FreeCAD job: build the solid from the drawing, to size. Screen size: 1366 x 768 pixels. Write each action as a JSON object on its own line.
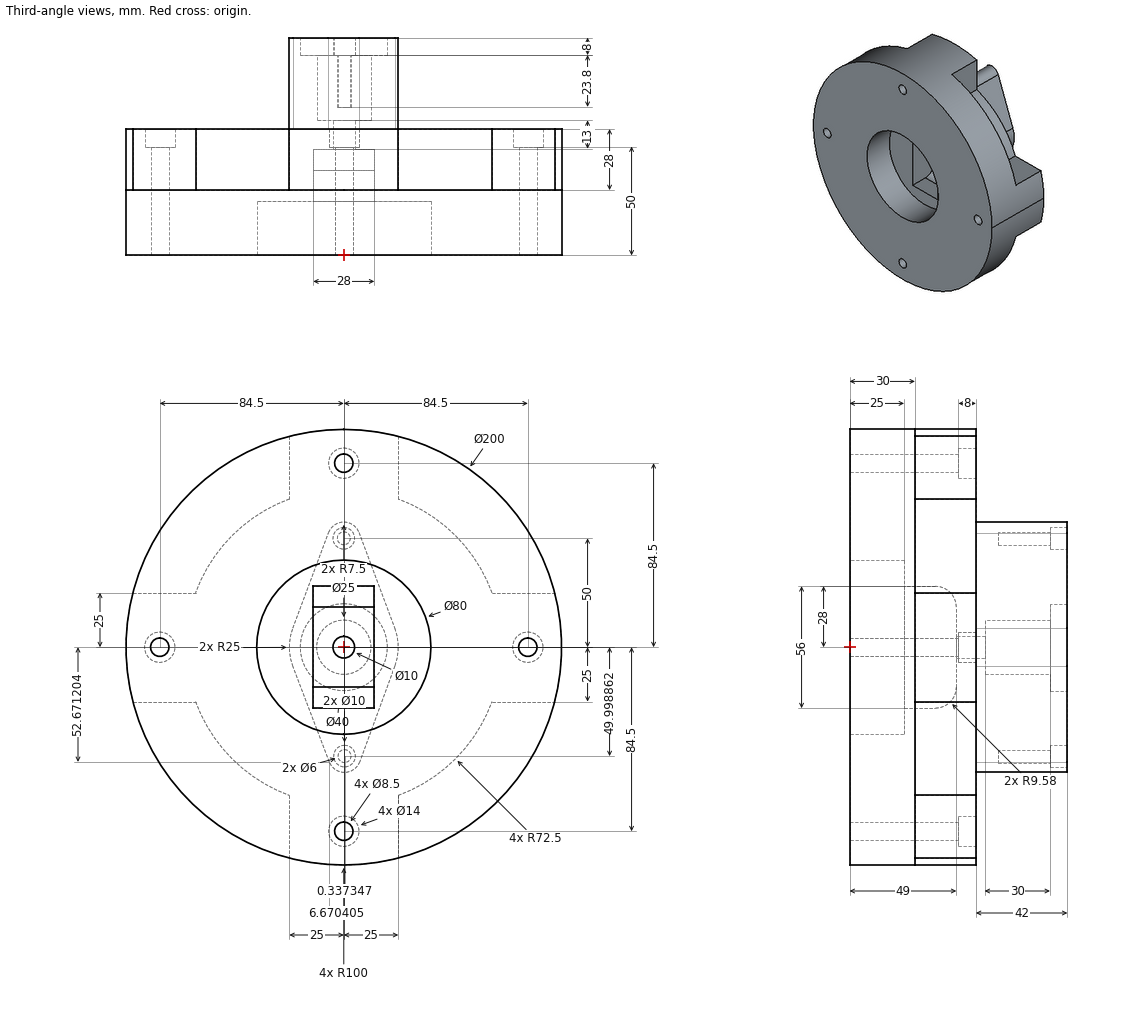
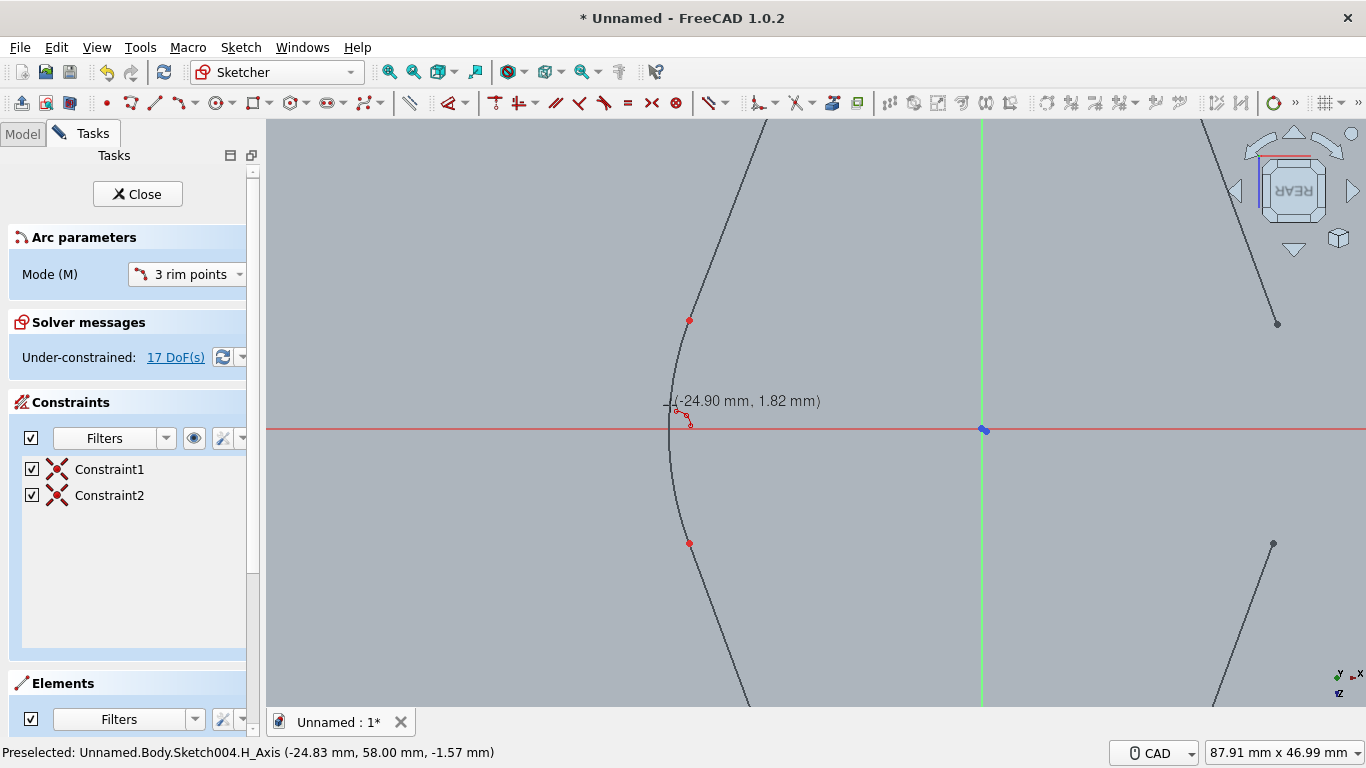
{"action": "scroll", "coordinate": [671, 408], "scroll_direction": "down", "scroll_amount": 7}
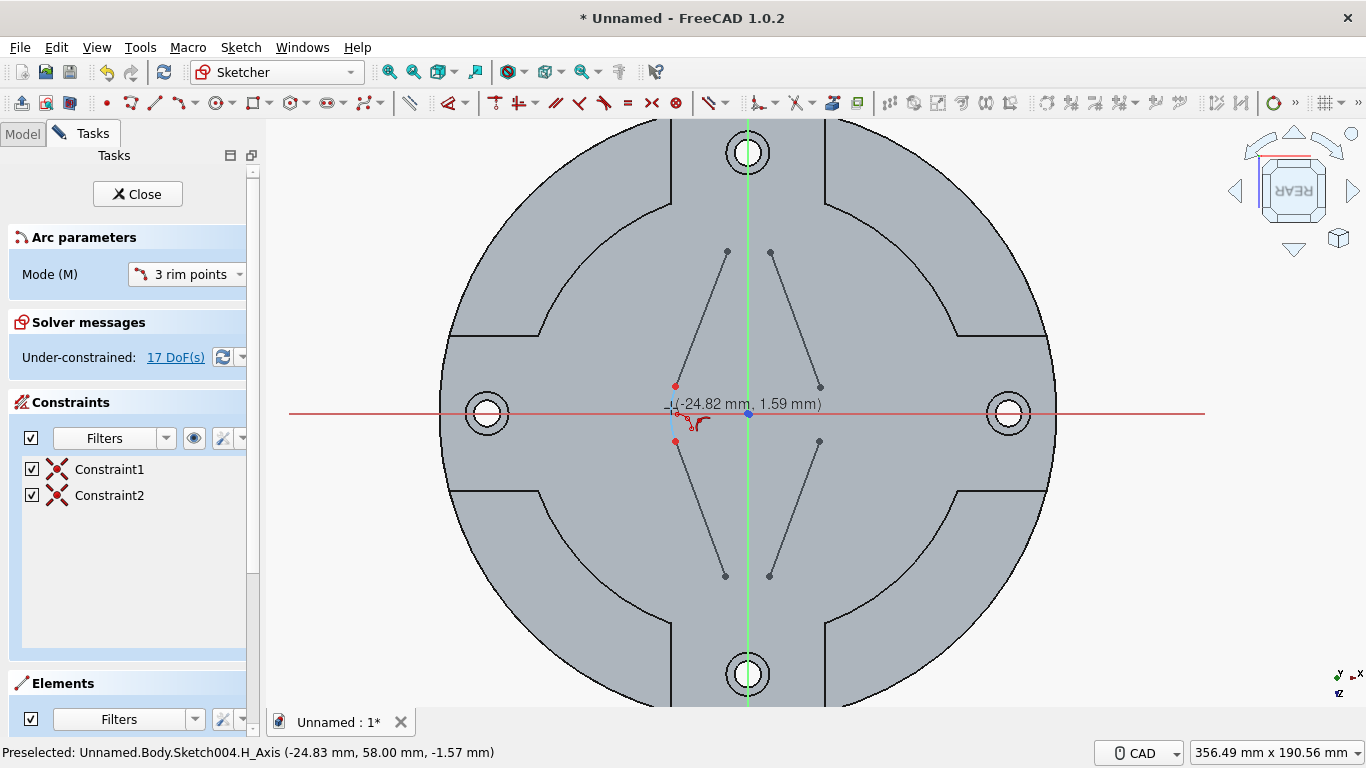
{"action": "left_click", "coordinate": [726, 577]}
{"action": "left_click", "coordinate": [770, 577]}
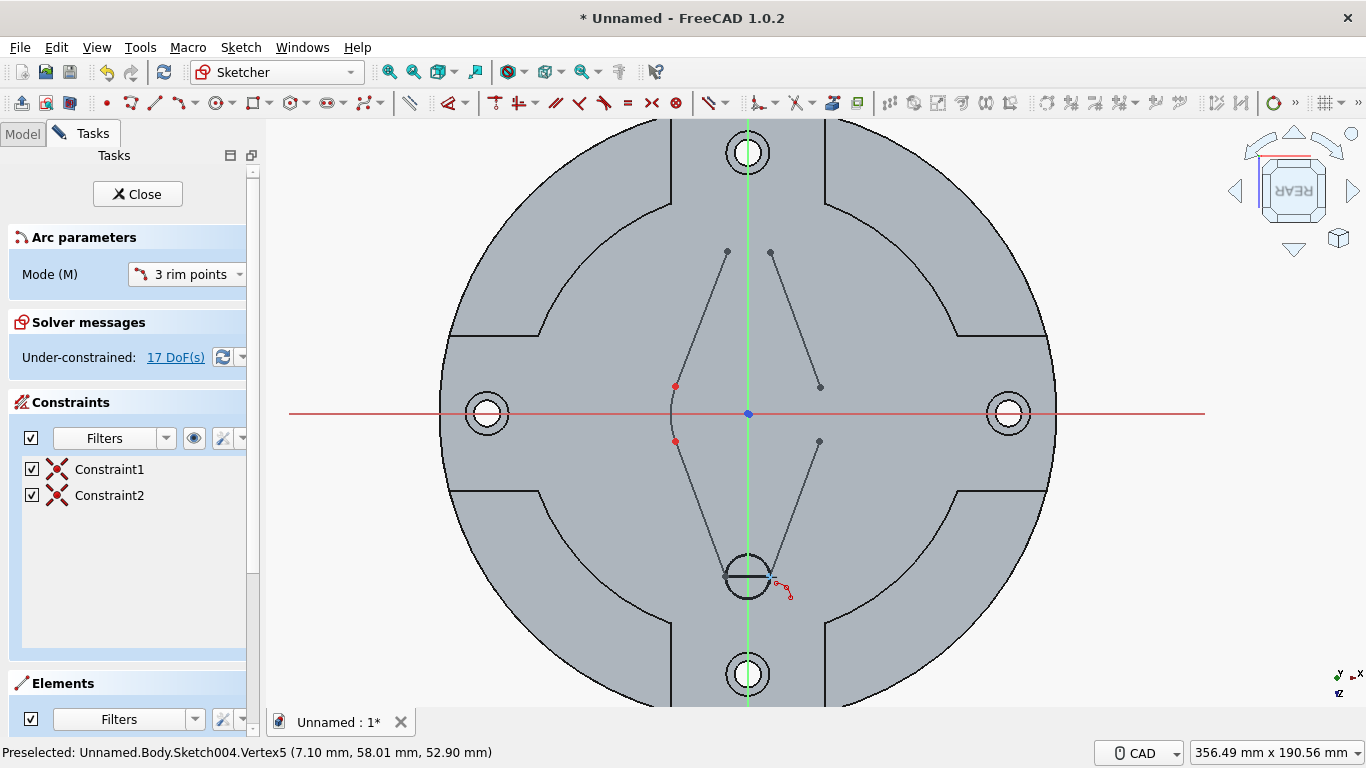
{"action": "scroll", "coordinate": [737, 588], "scroll_direction": "up", "scroll_amount": 2}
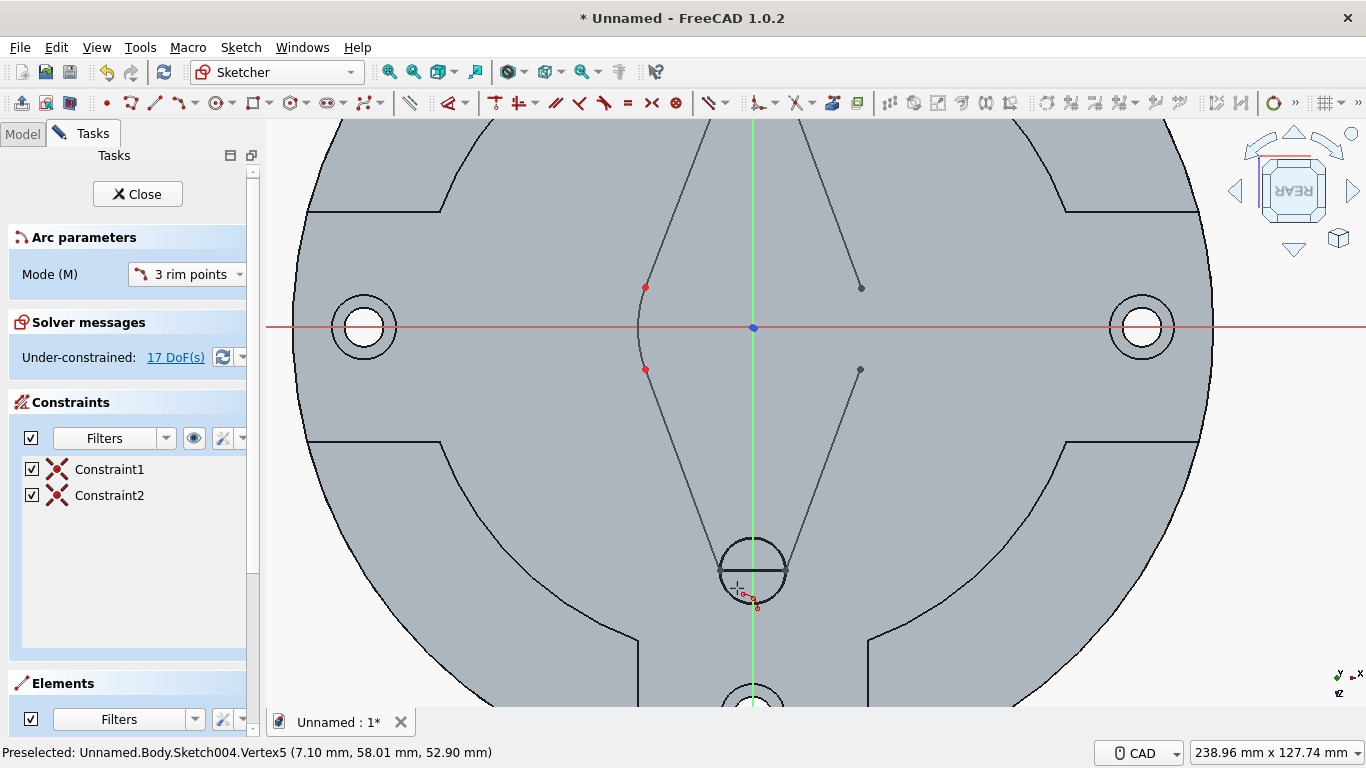
{"action": "left_click", "coordinate": [737, 588]}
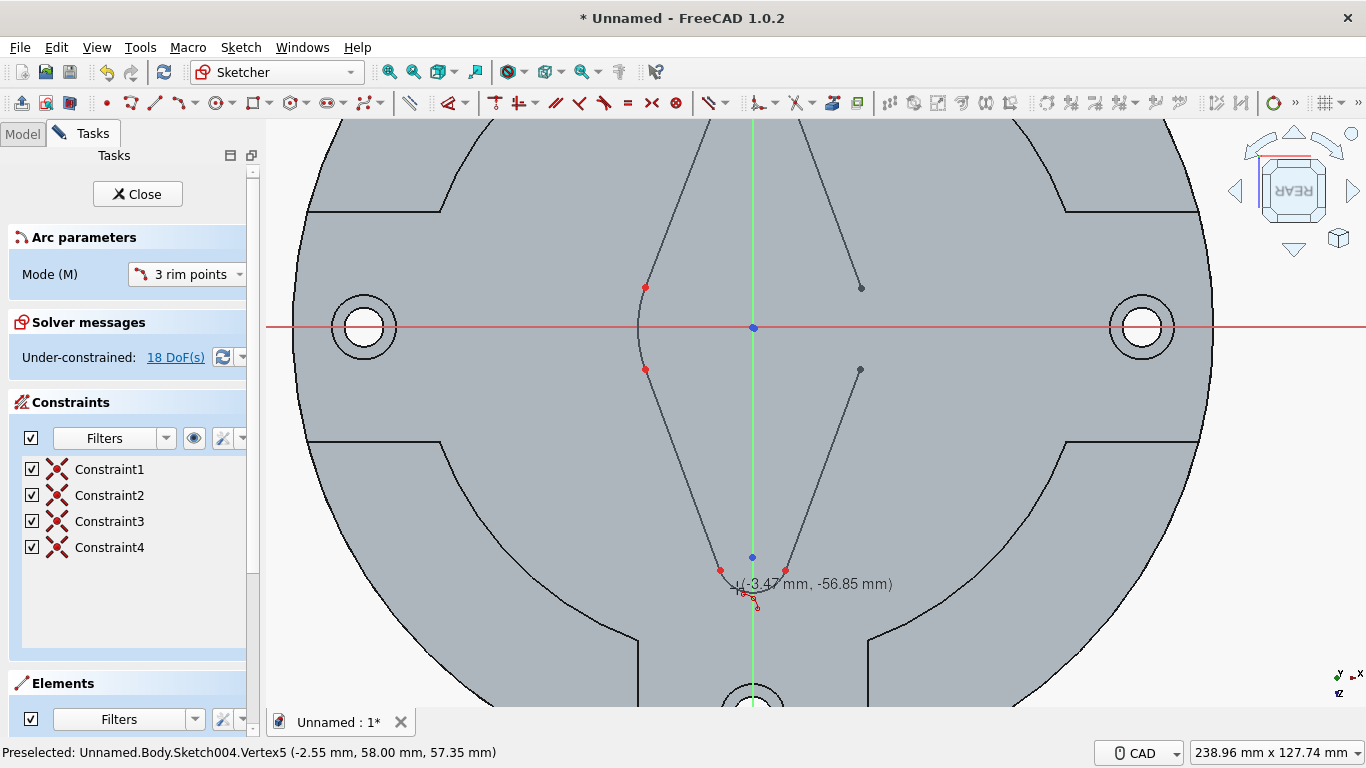
{"action": "left_click", "coordinate": [860, 369]}
{"action": "left_click", "coordinate": [862, 289]}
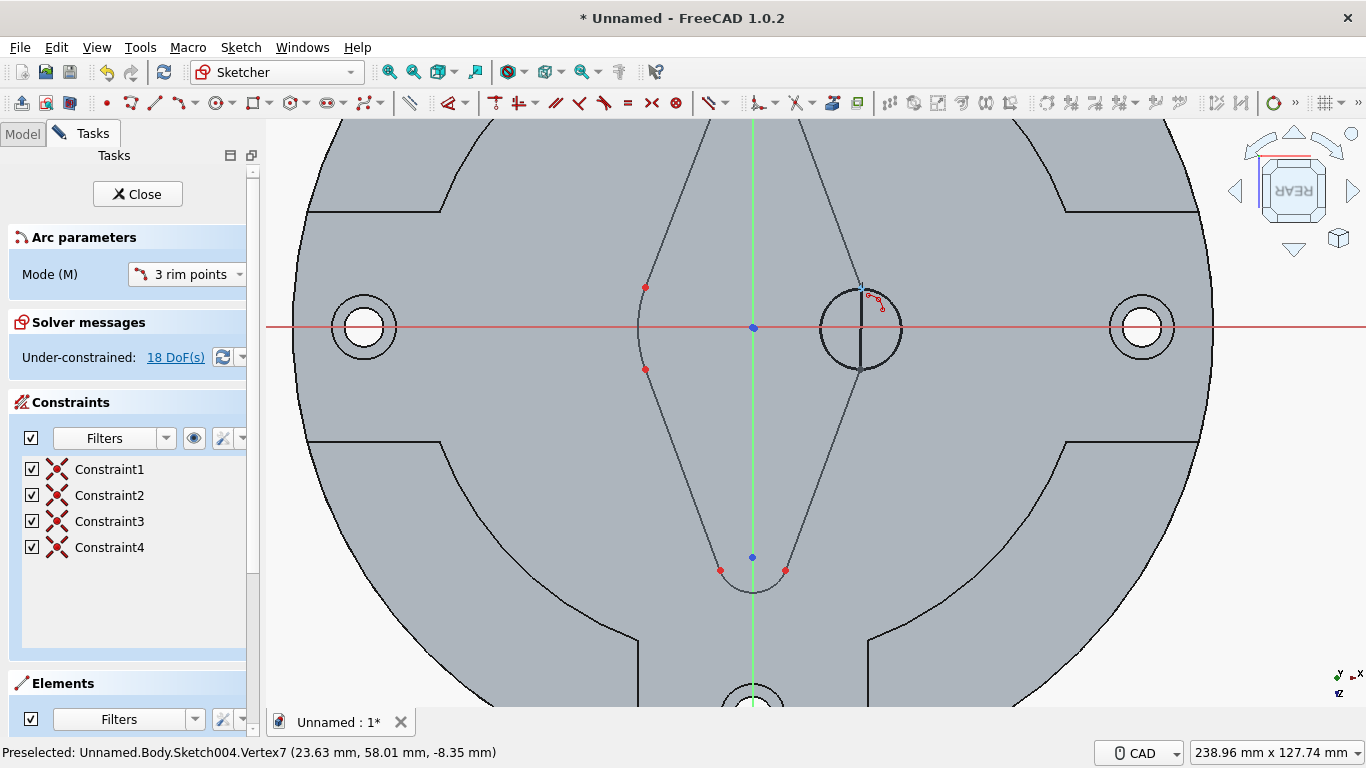
{"action": "scroll", "coordinate": [868, 336], "scroll_direction": "up", "scroll_amount": 5}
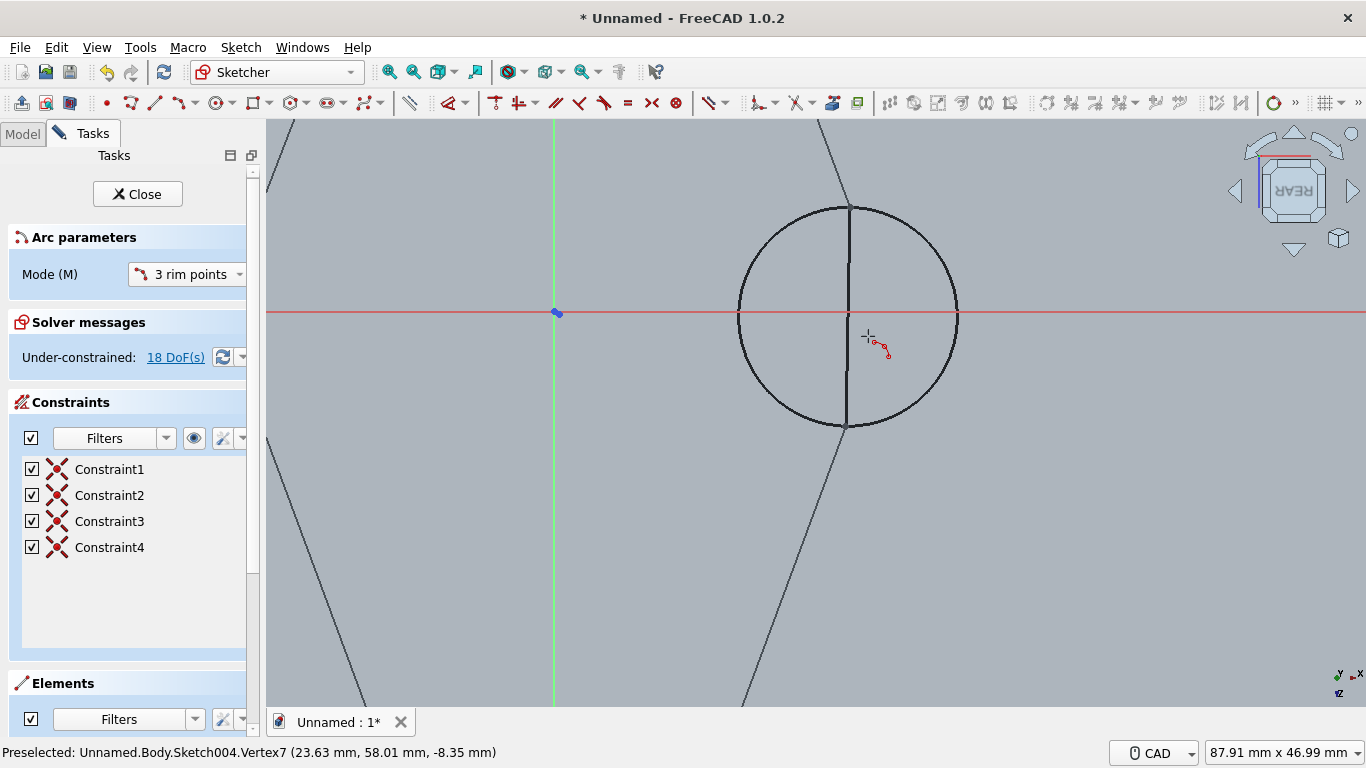
{"action": "left_click", "coordinate": [866, 335]}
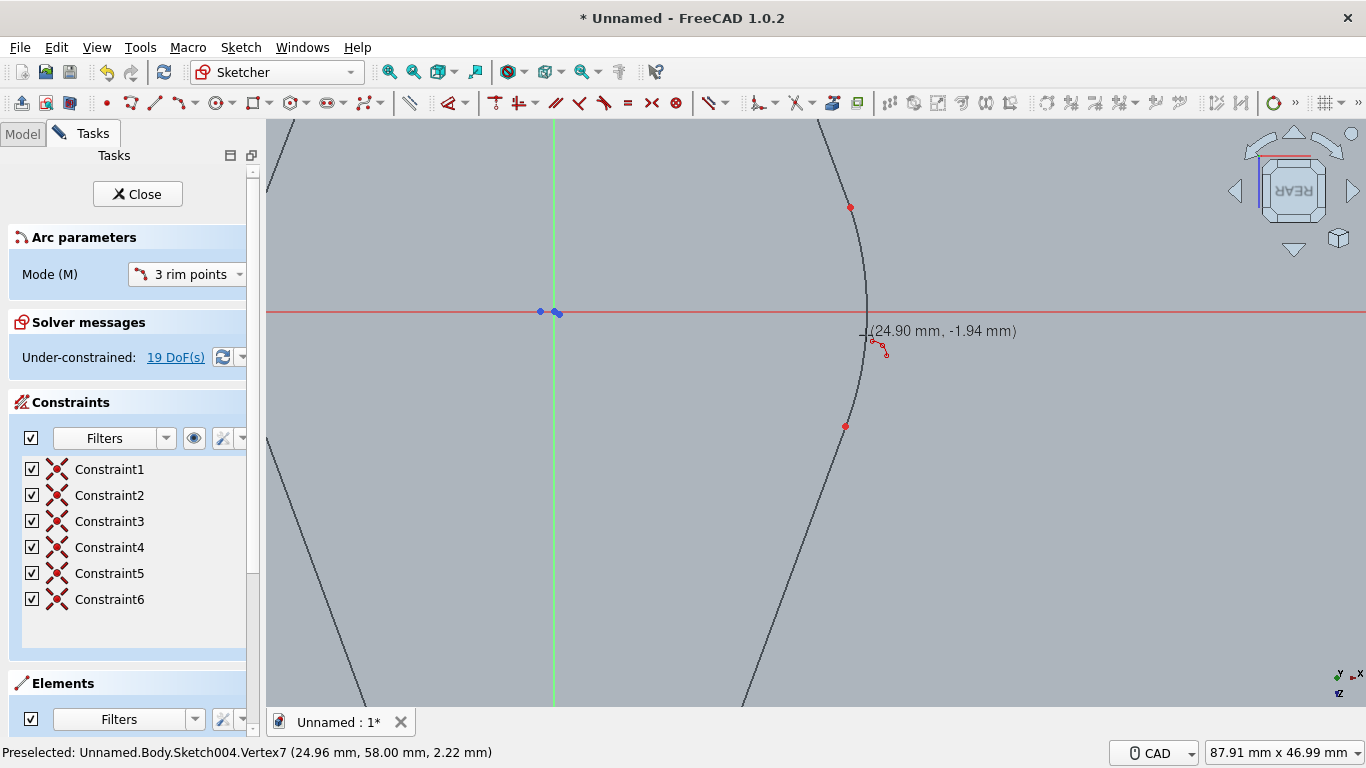
{"action": "scroll", "coordinate": [811, 446], "scroll_direction": "down", "scroll_amount": 7}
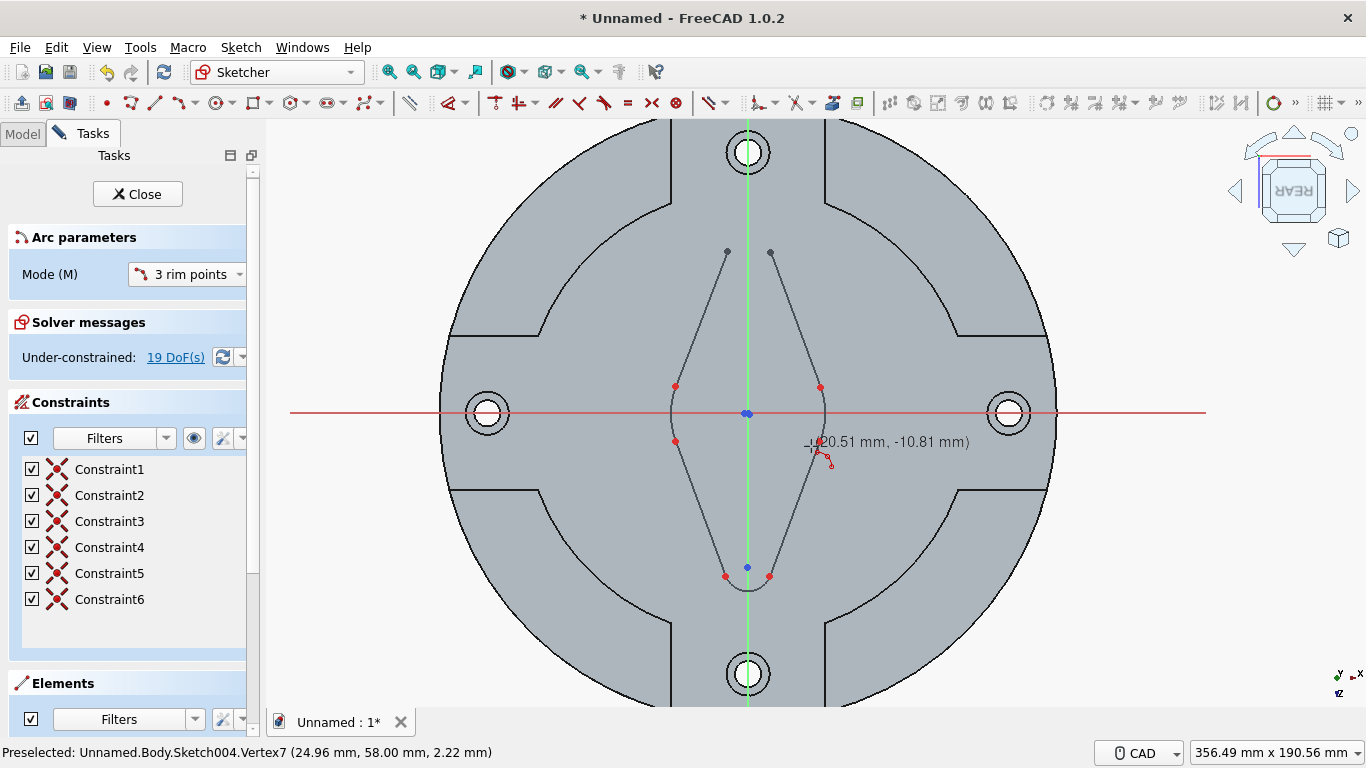
{"action": "left_click", "coordinate": [771, 253]}
{"action": "left_click", "coordinate": [728, 252]}